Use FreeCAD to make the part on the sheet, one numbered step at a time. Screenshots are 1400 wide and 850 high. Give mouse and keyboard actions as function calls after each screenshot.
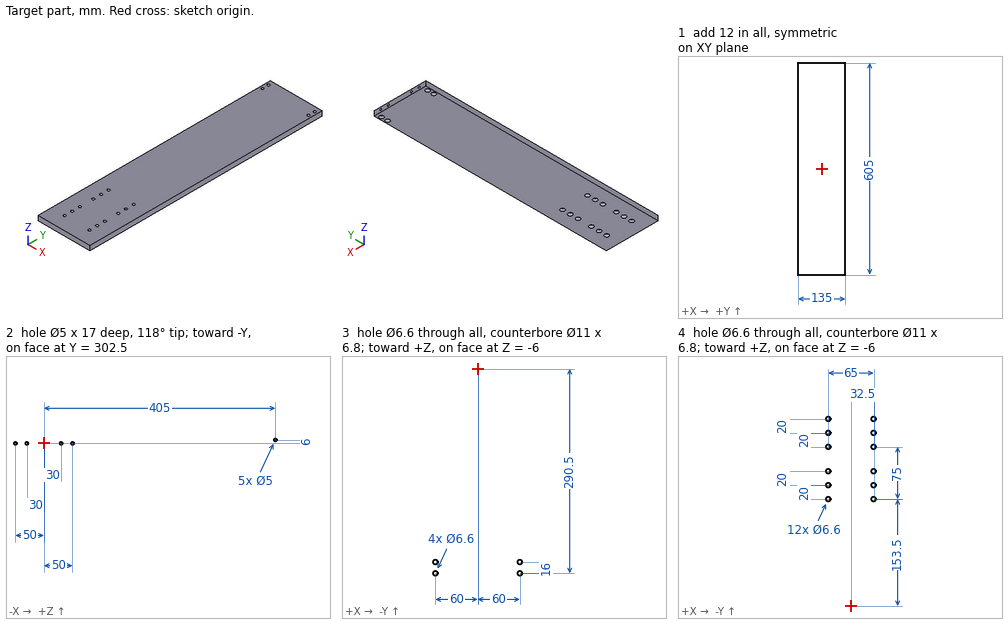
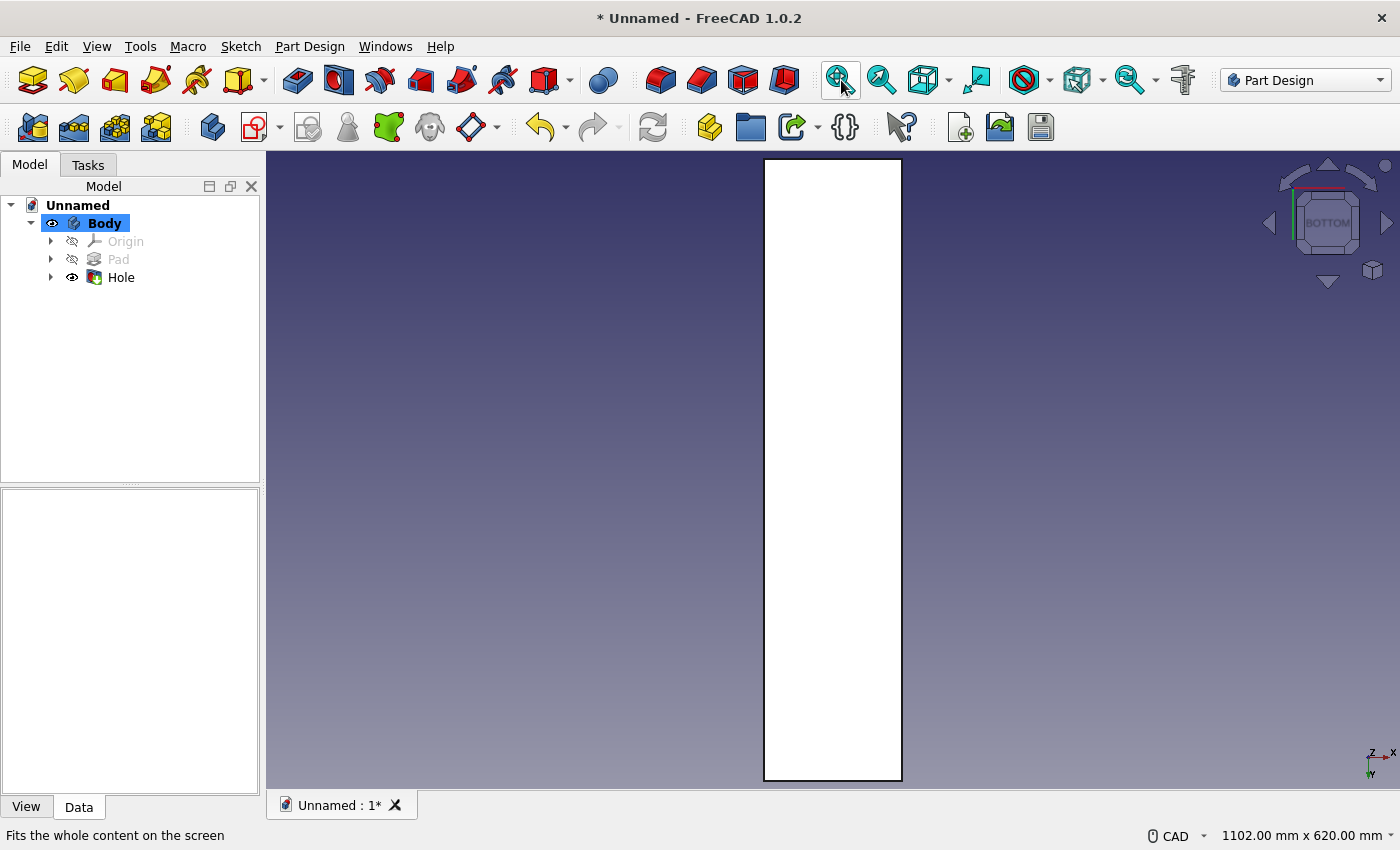
click(833, 647)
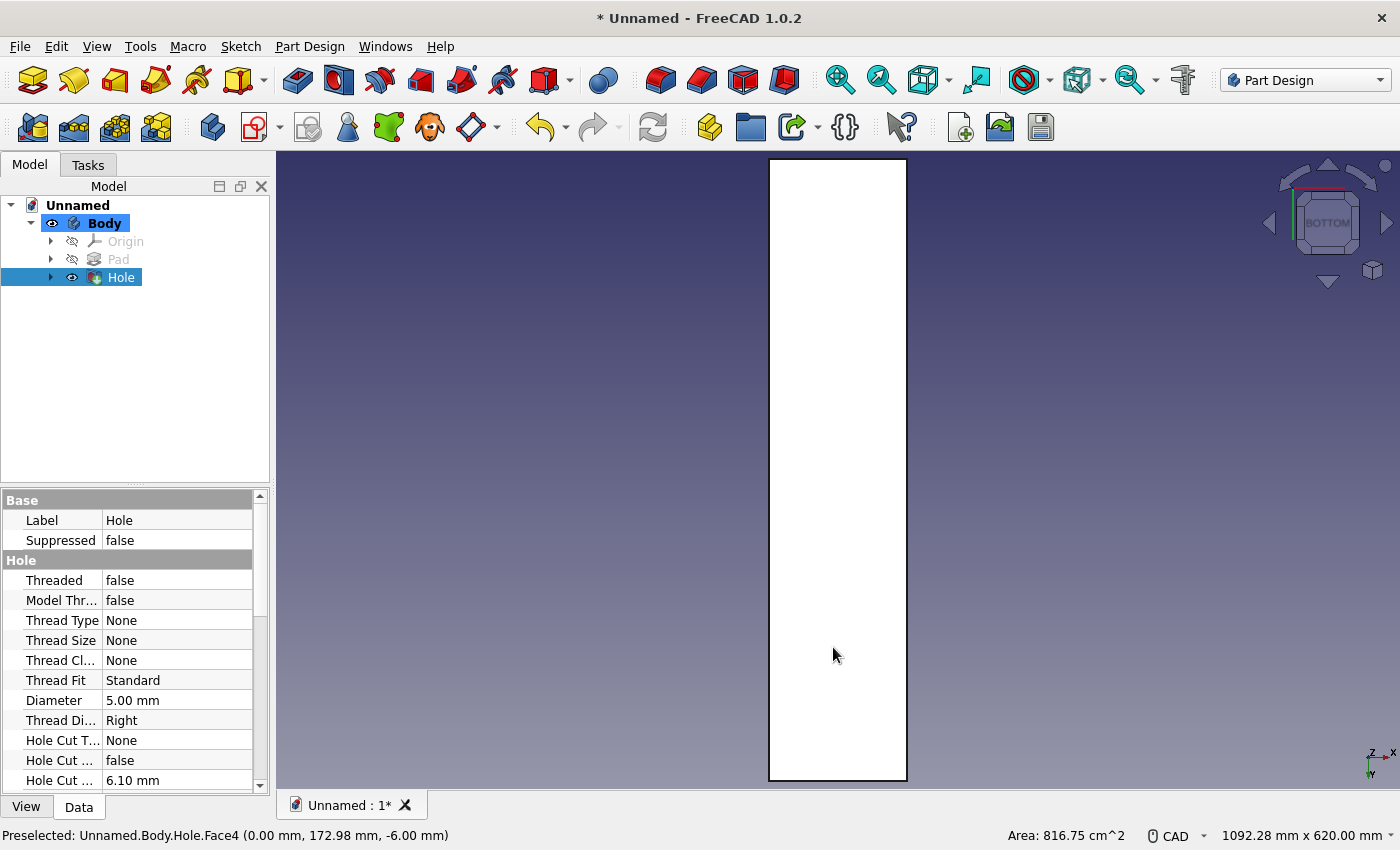
click(254, 128)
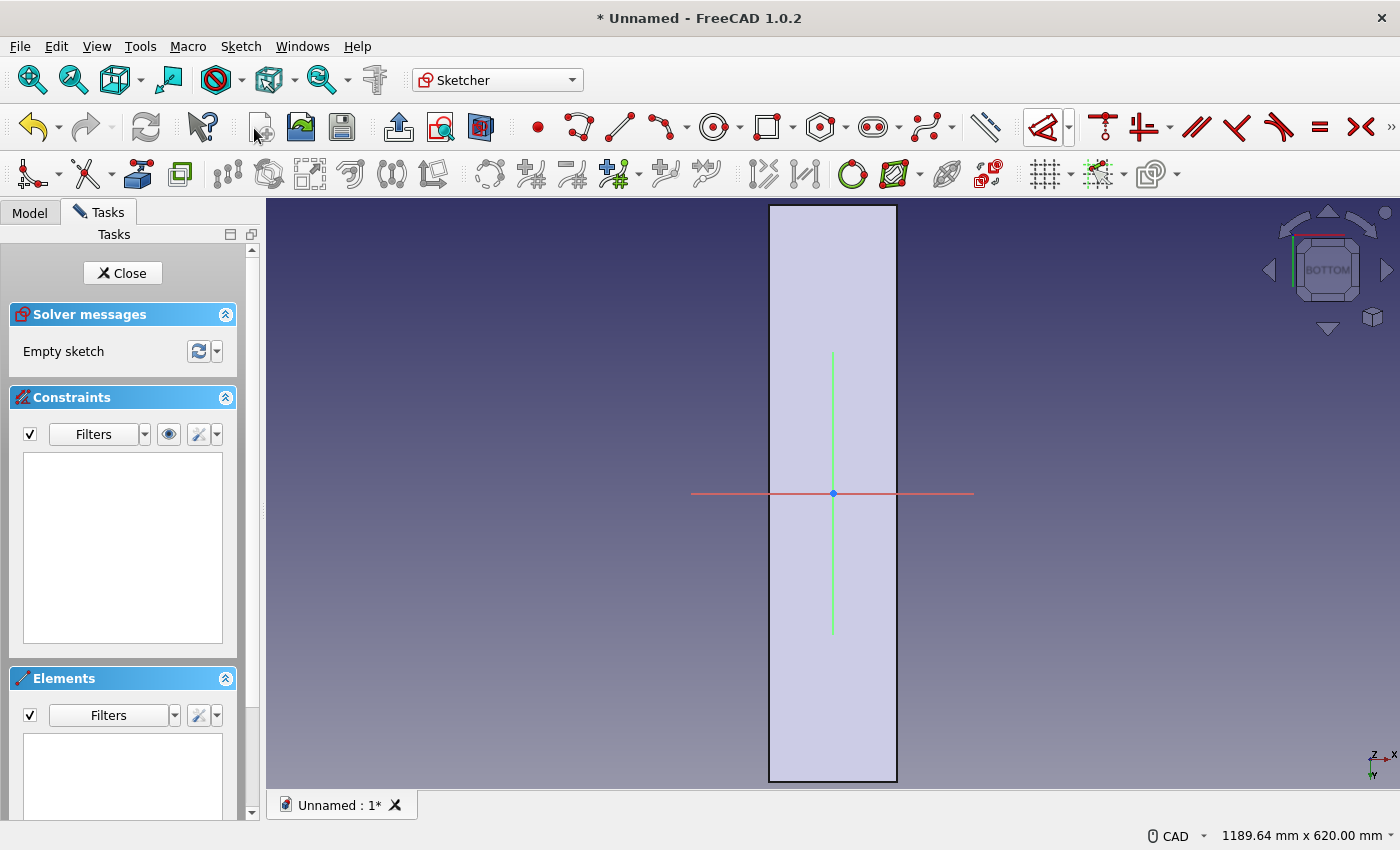
scroll(455, 226, down, 1)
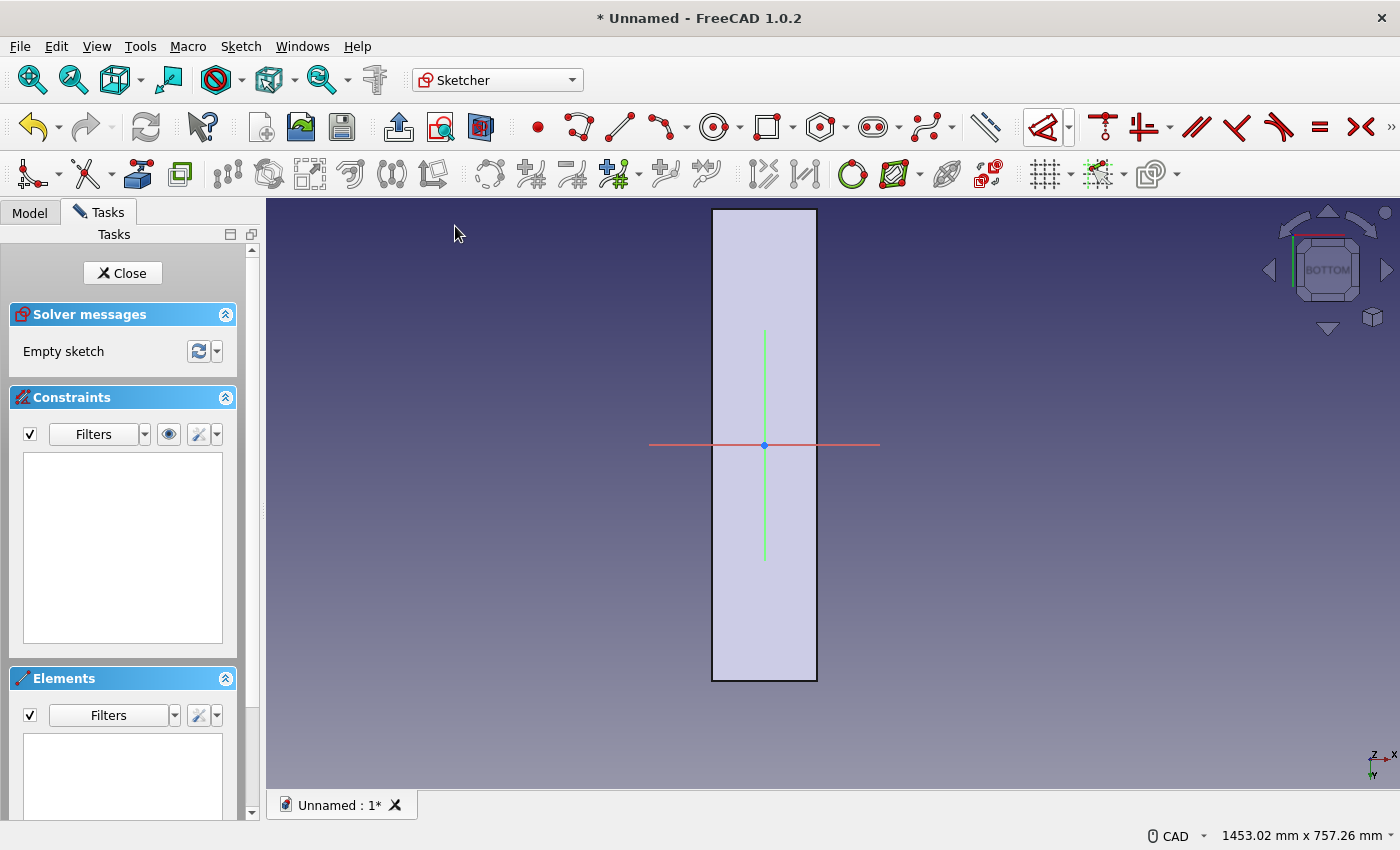
scroll(765, 694, up, 2)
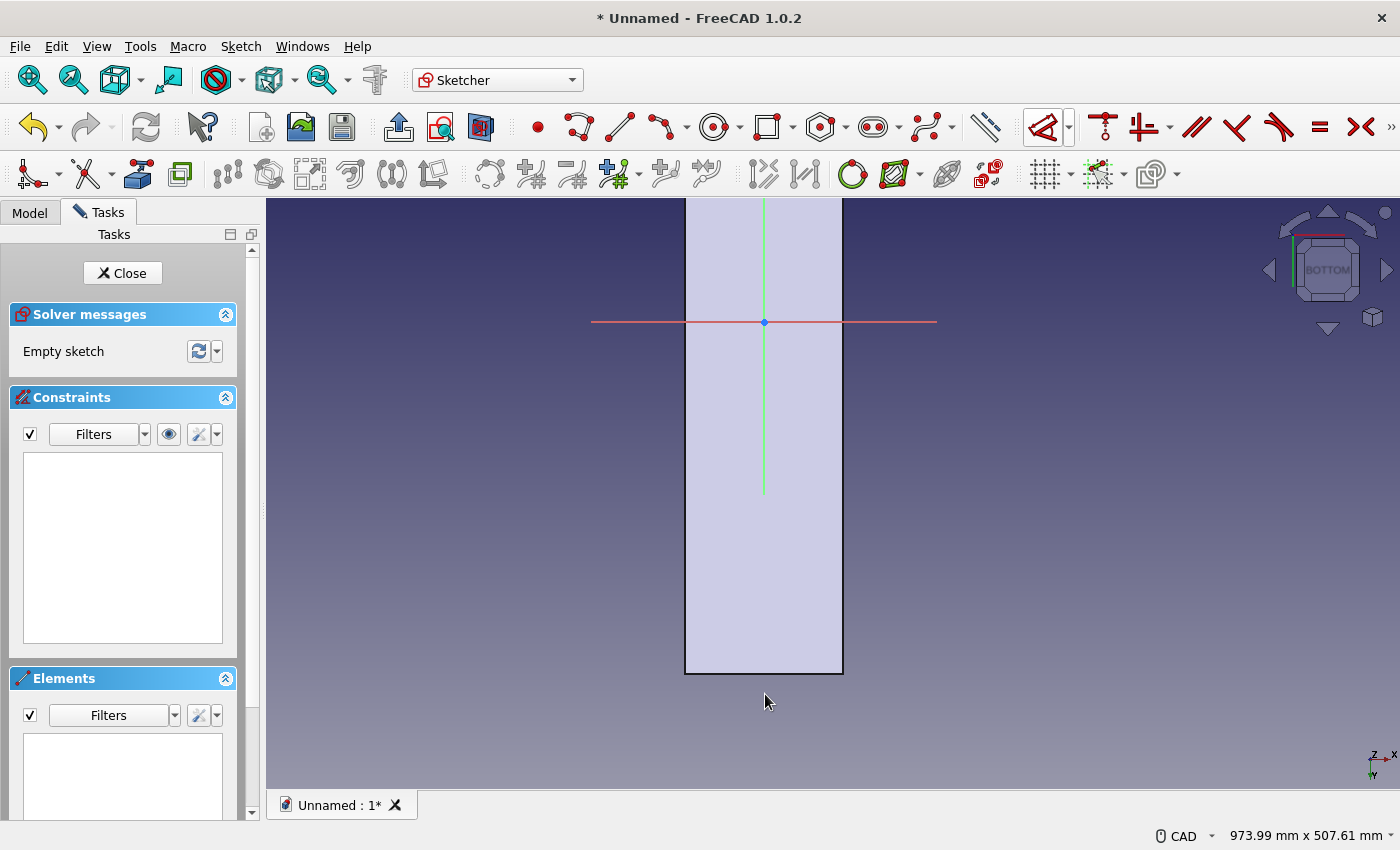
click(714, 128)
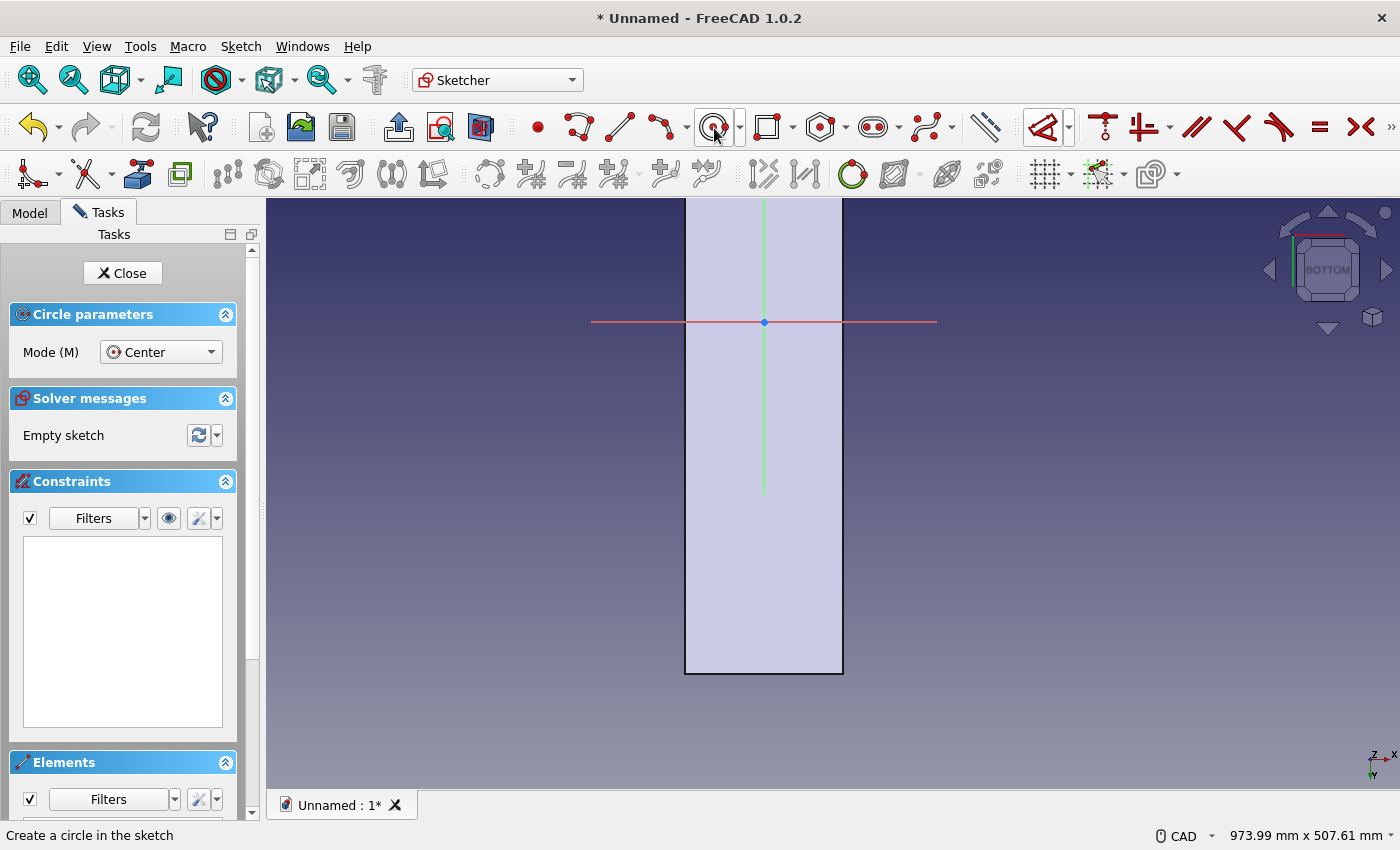
scroll(834, 660, up, 9)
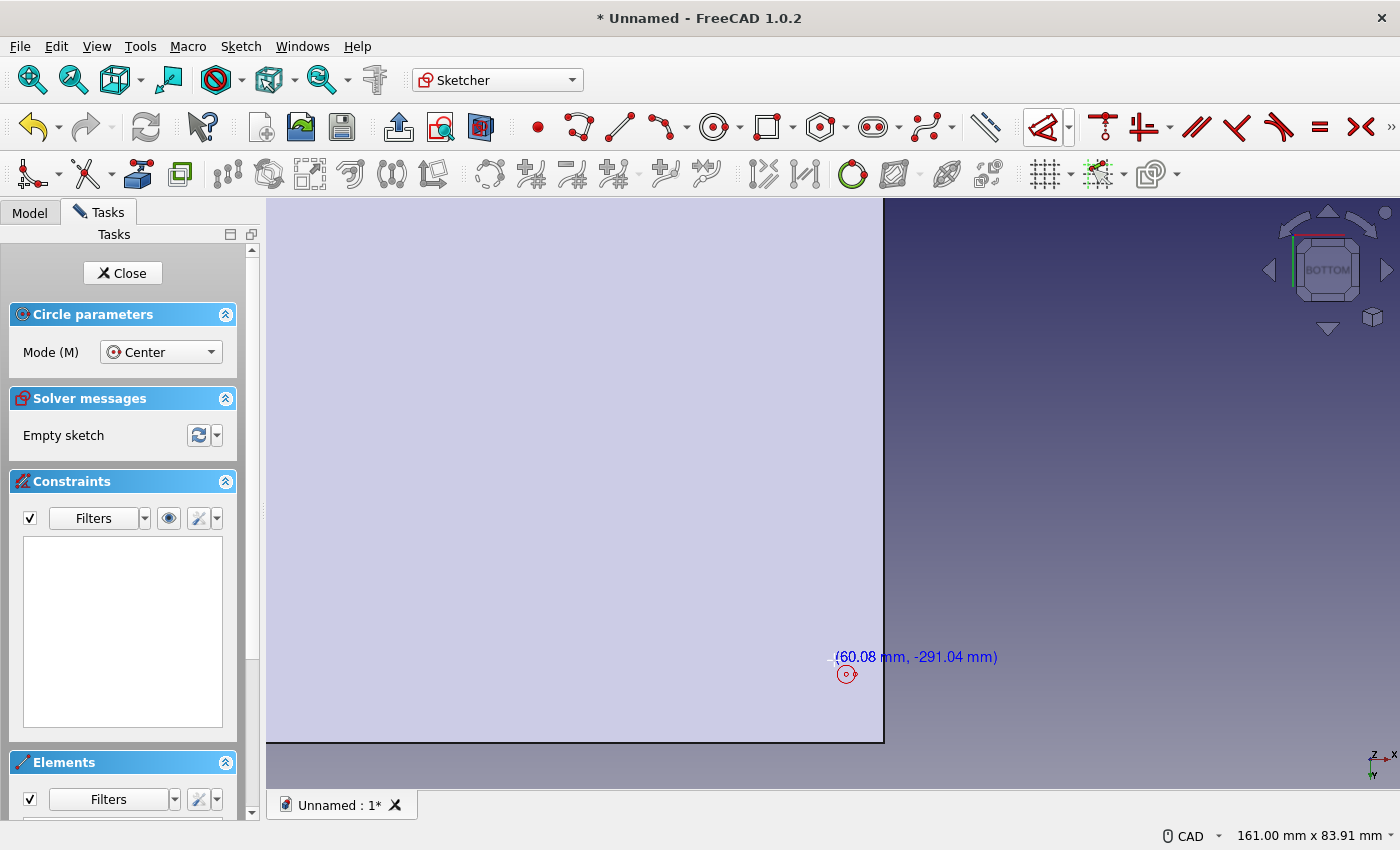
scroll(835, 661, down, 9)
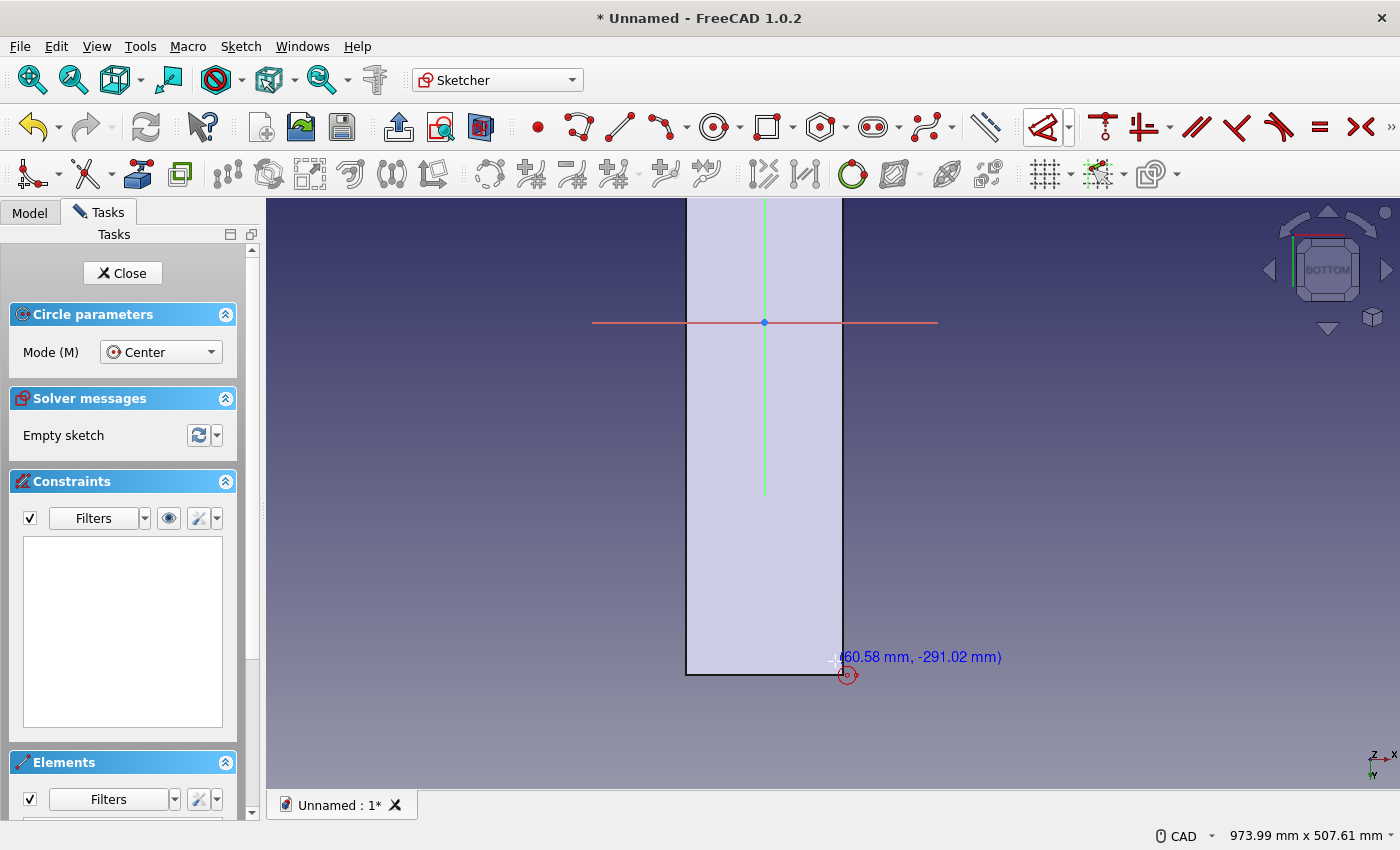
click(835, 661)
move(837, 658)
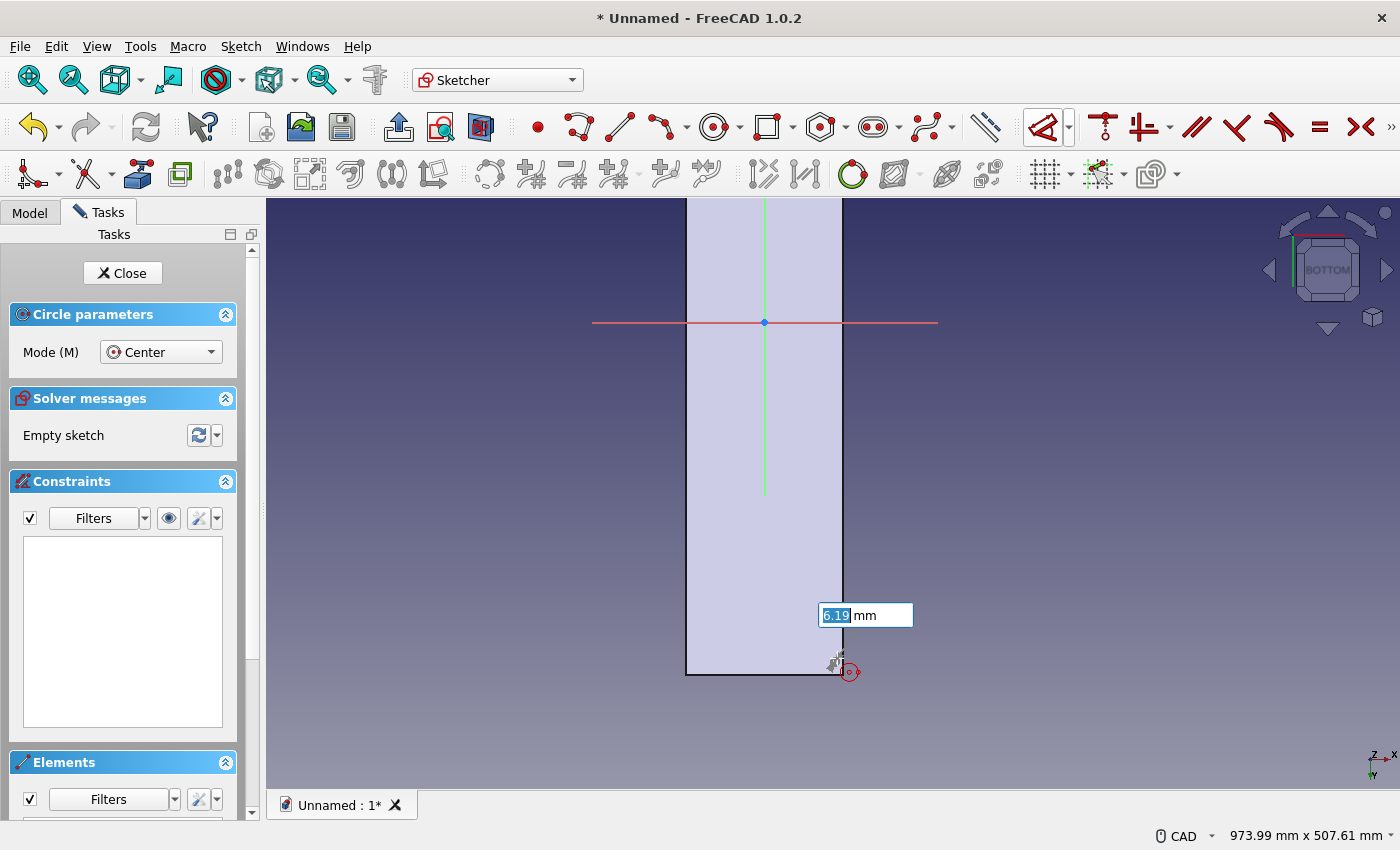
text(6.6)
key(Return)